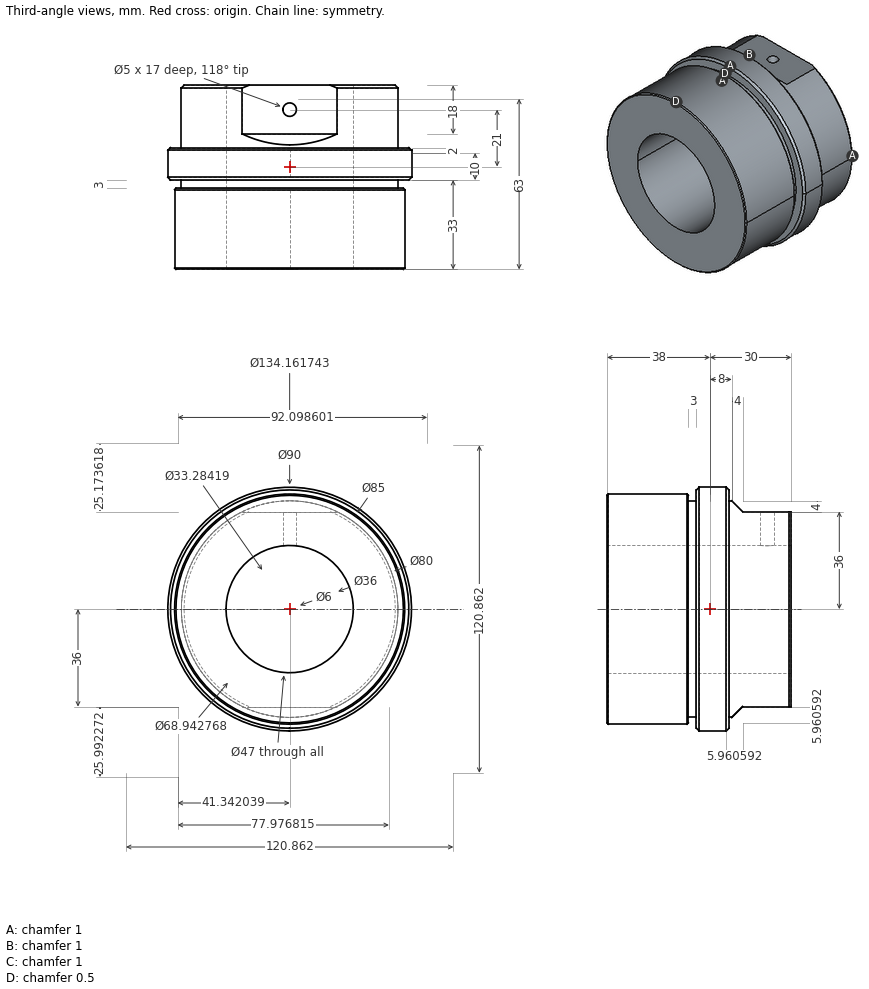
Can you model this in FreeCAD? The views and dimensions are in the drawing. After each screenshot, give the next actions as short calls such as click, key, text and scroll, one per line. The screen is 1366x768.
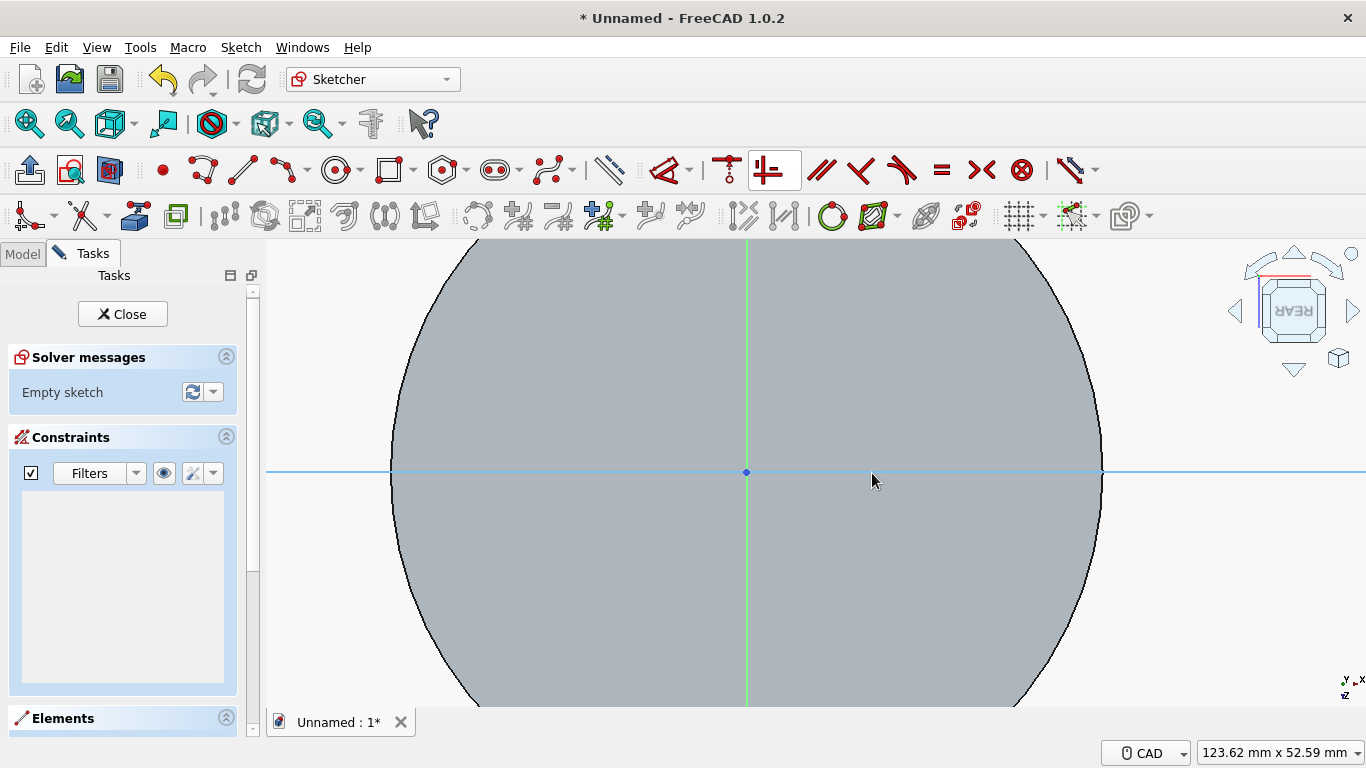
click(336, 170)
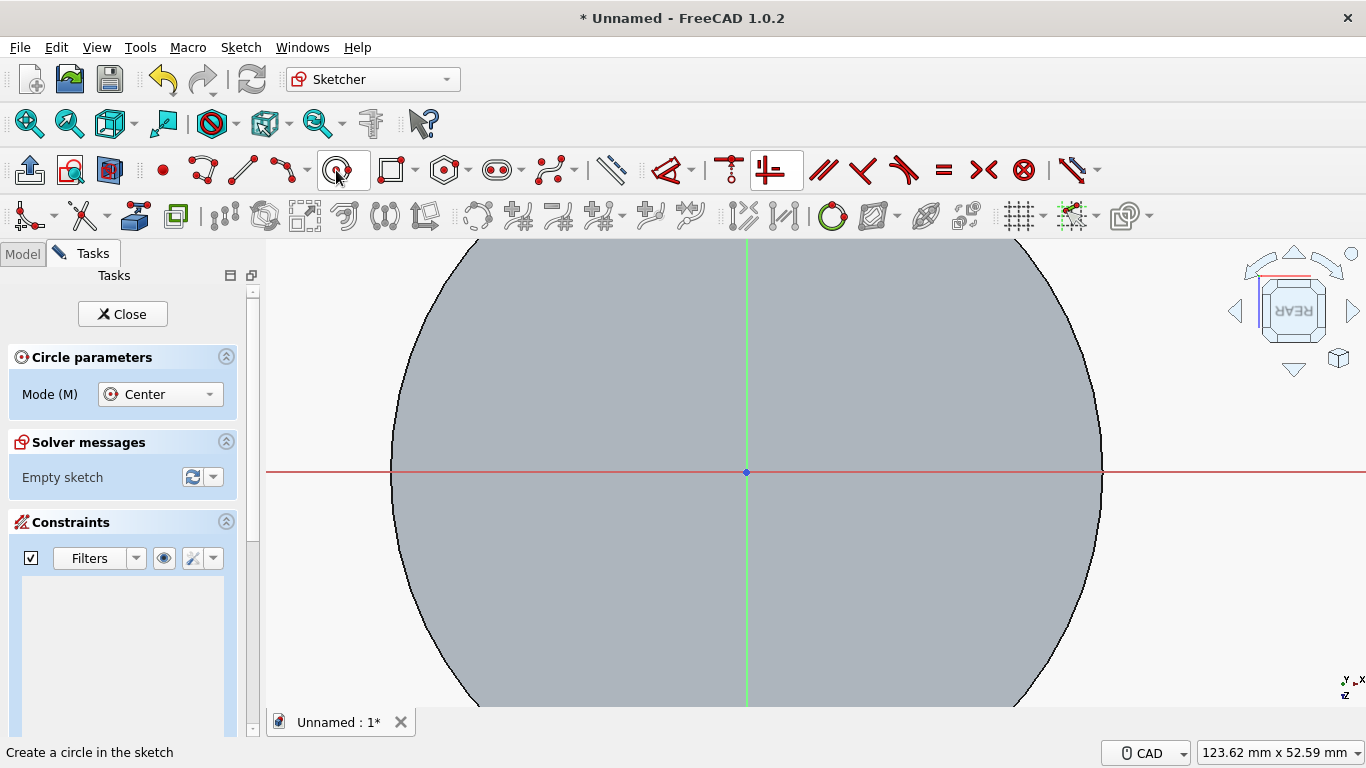
click(747, 472)
click(860, 359)
key(Escape)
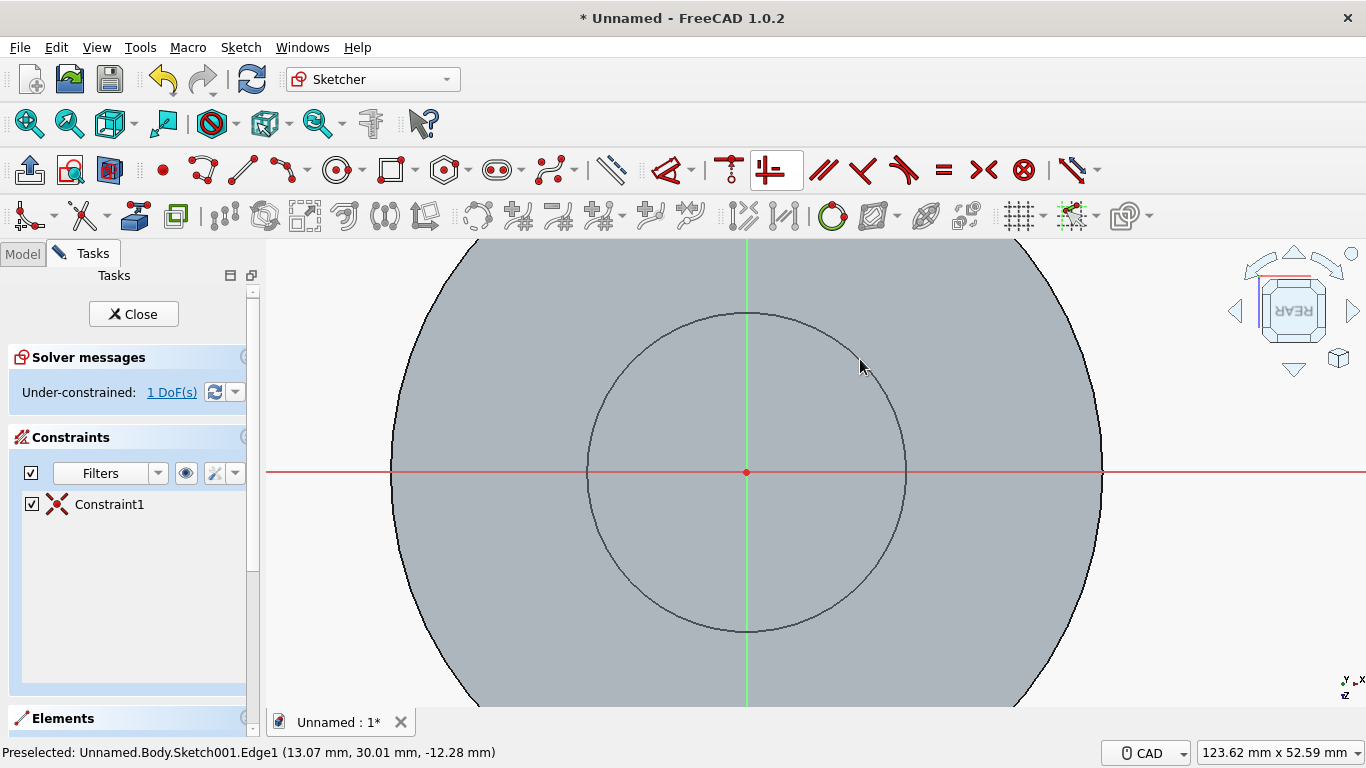
click(666, 170)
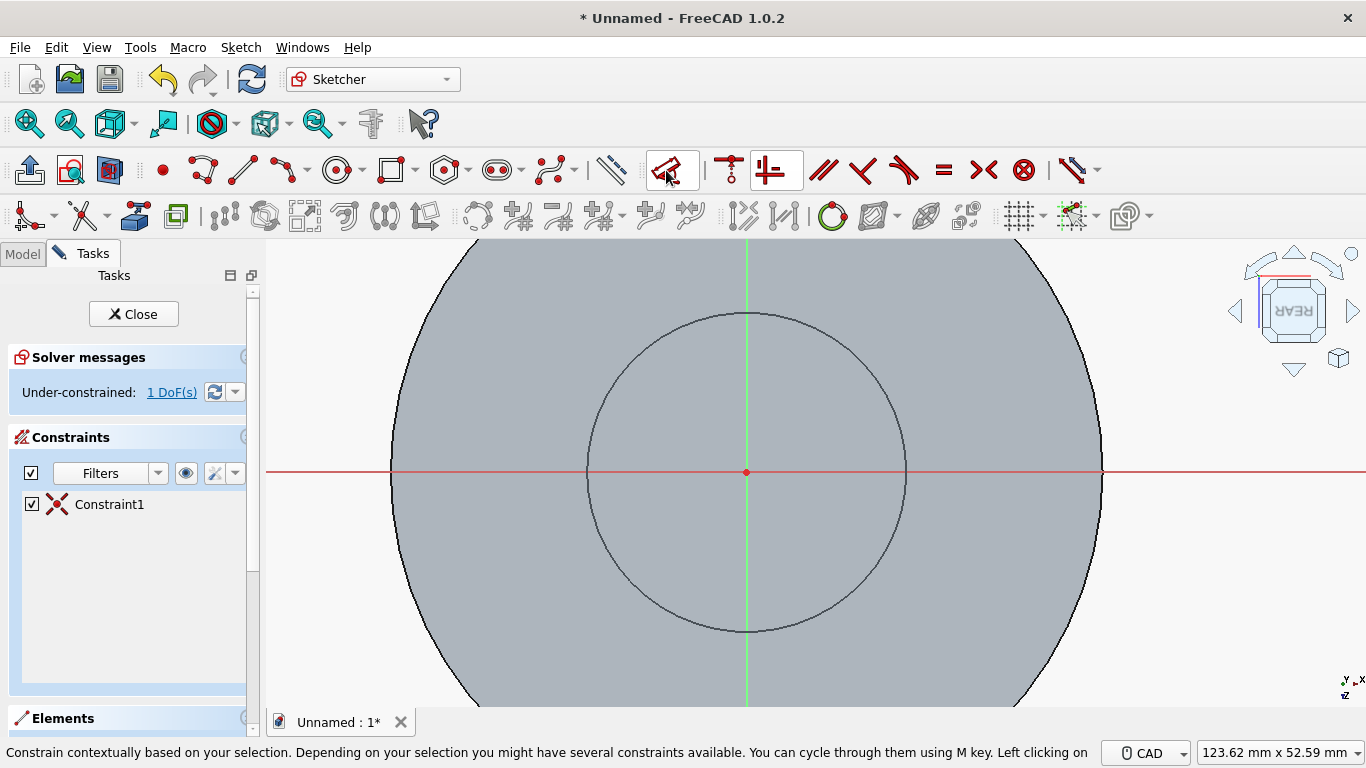
click(859, 359)
click(882, 336)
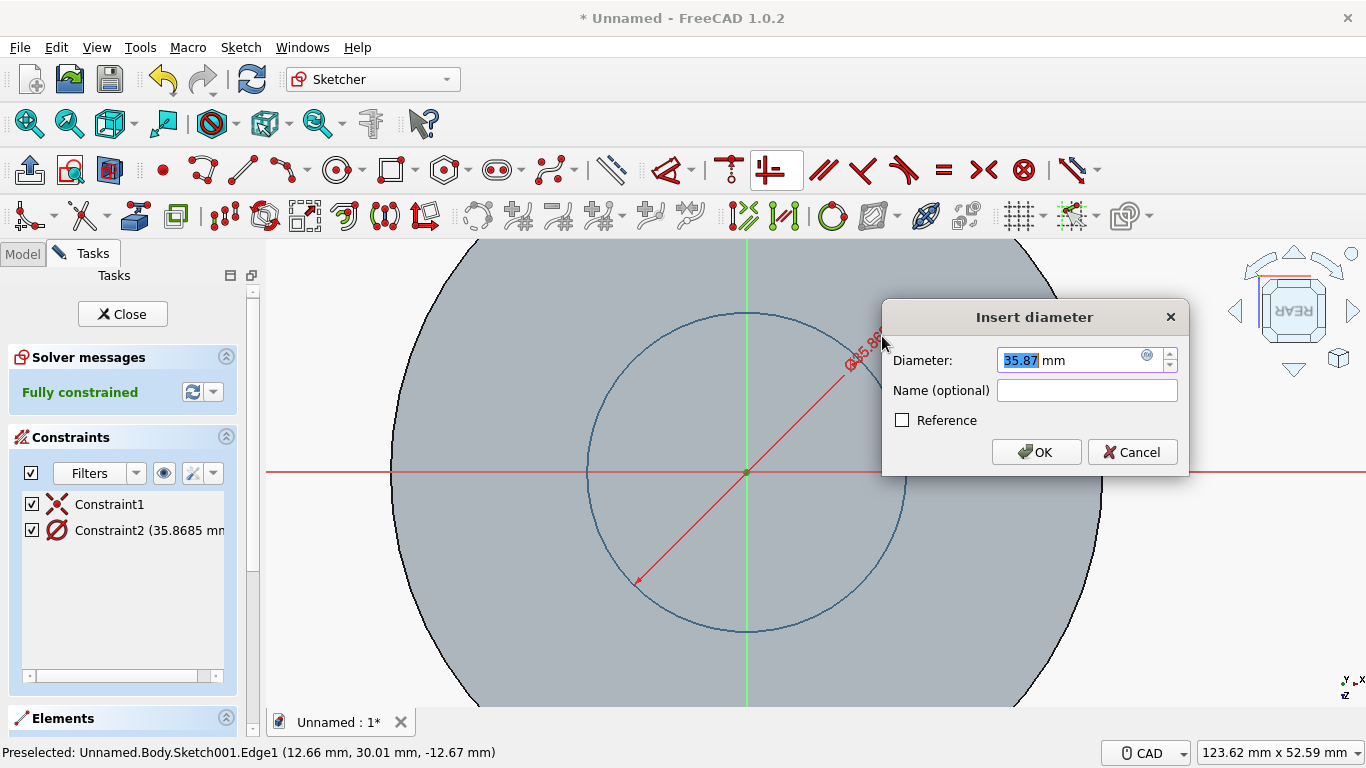
text(36)
key(Return)
key(Escape)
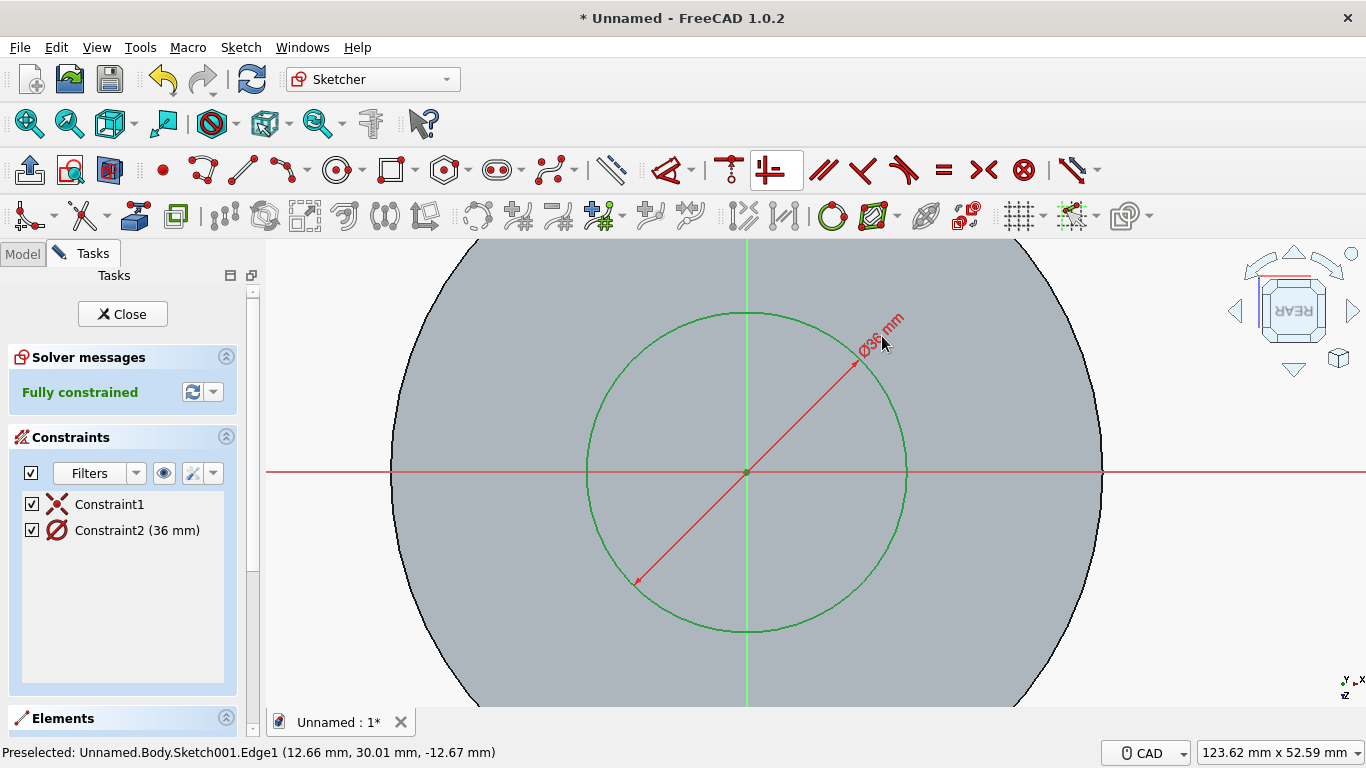
click(123, 314)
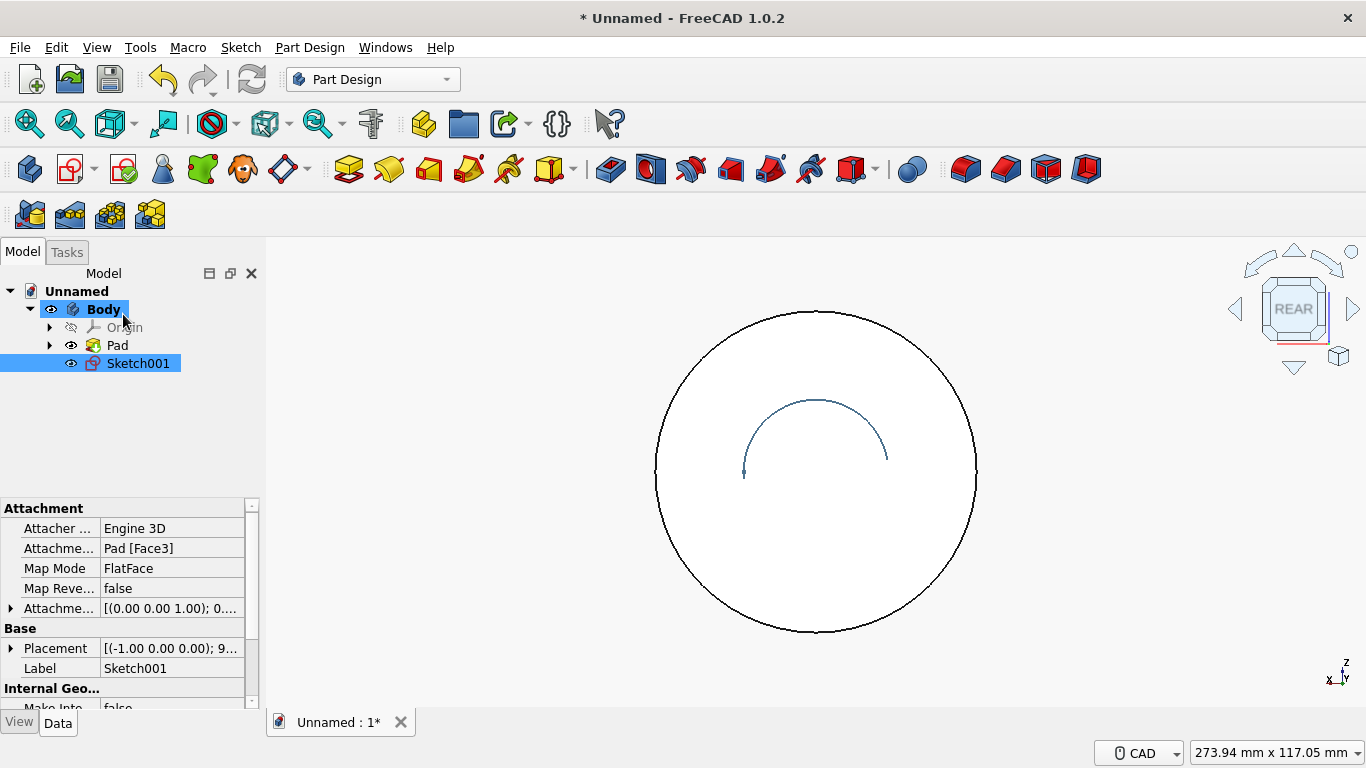
click(350, 170)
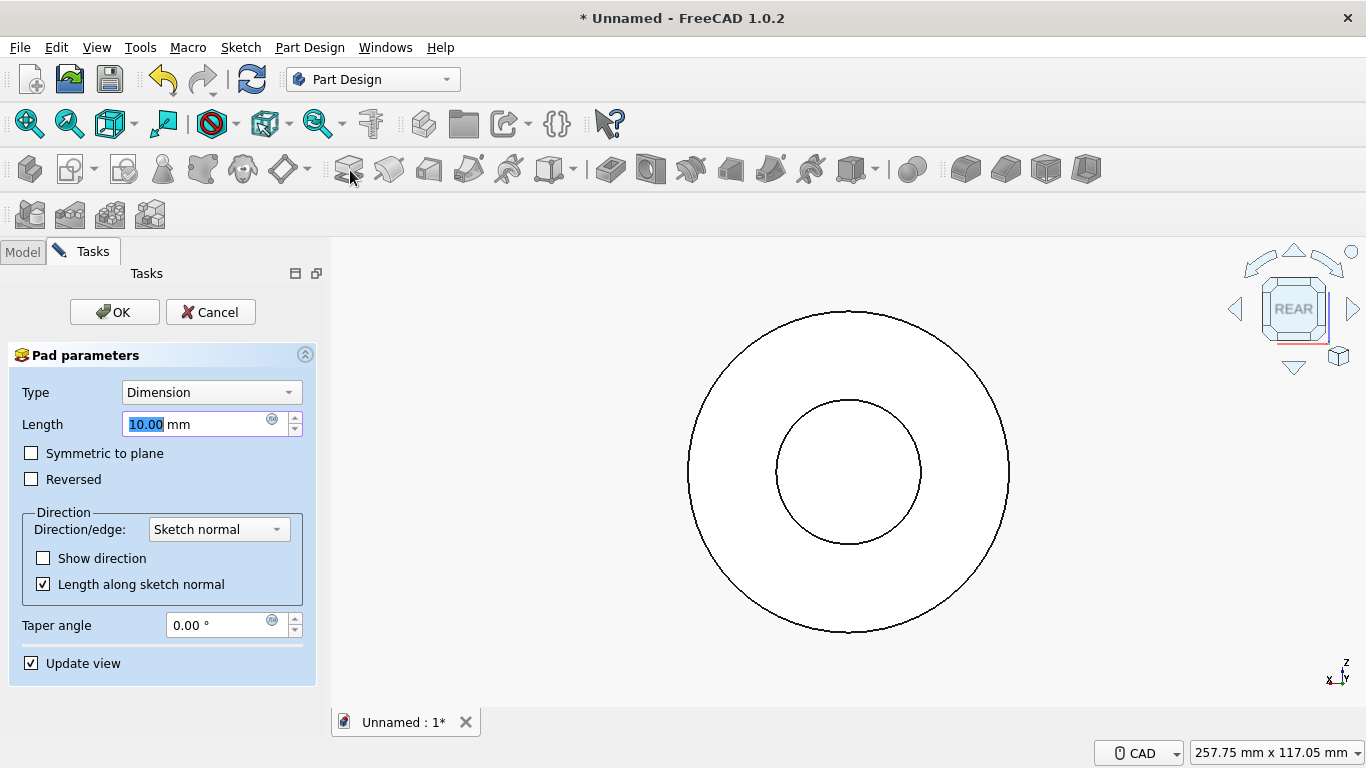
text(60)
key(Tab)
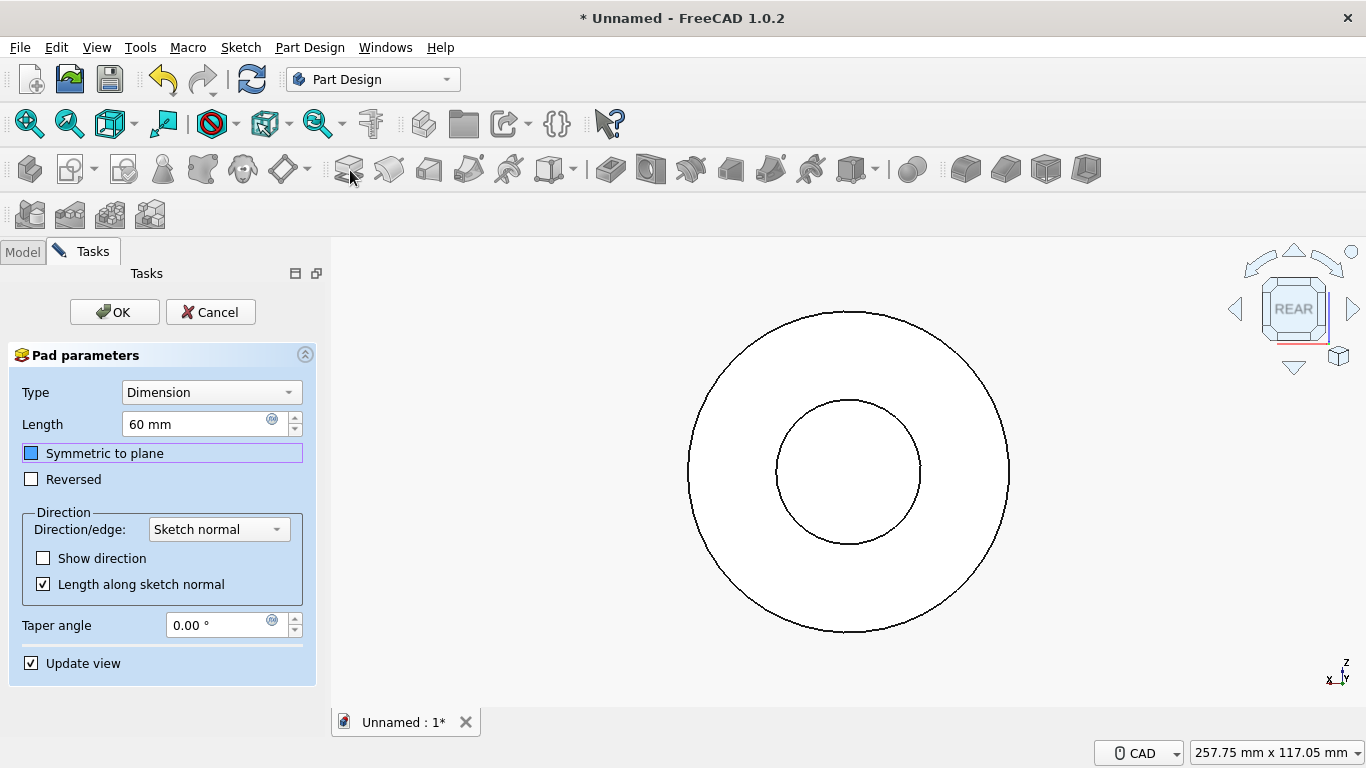
click(115, 312)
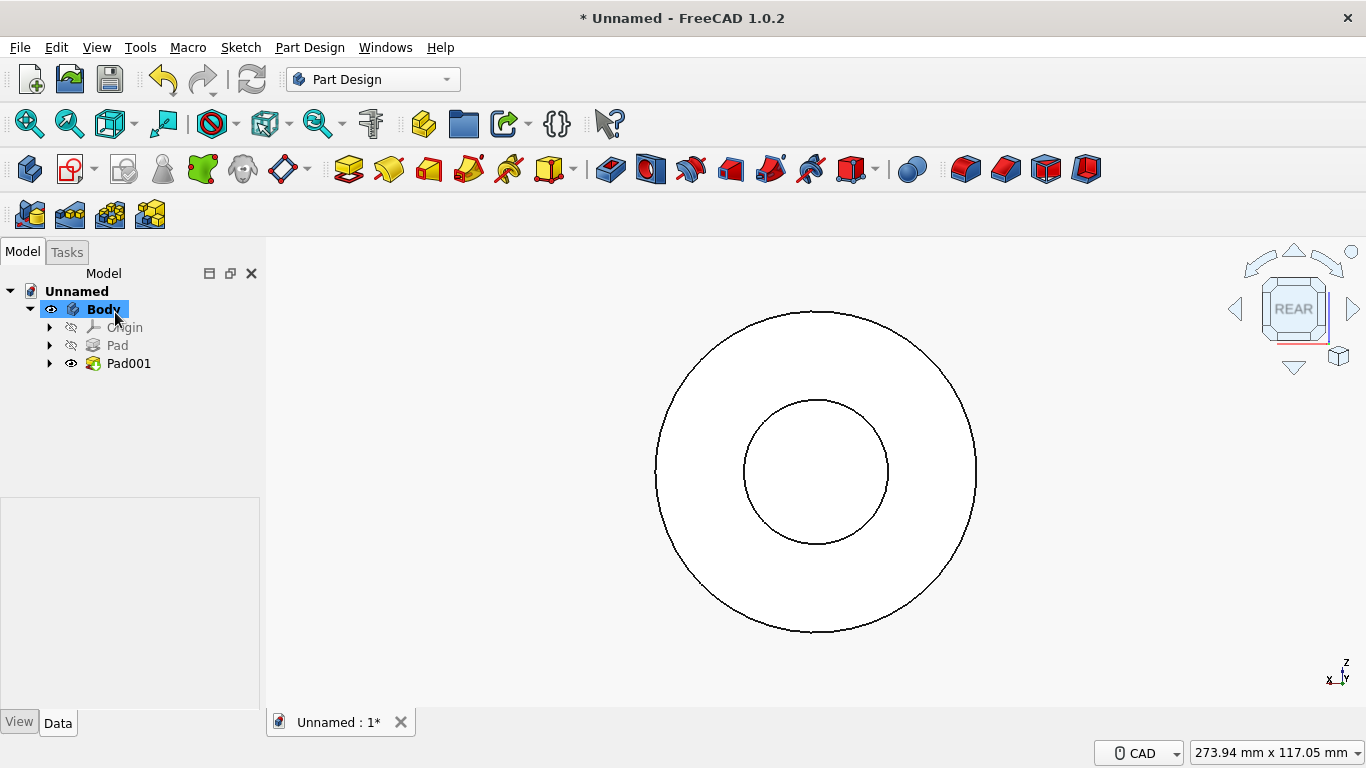
click(724, 563)